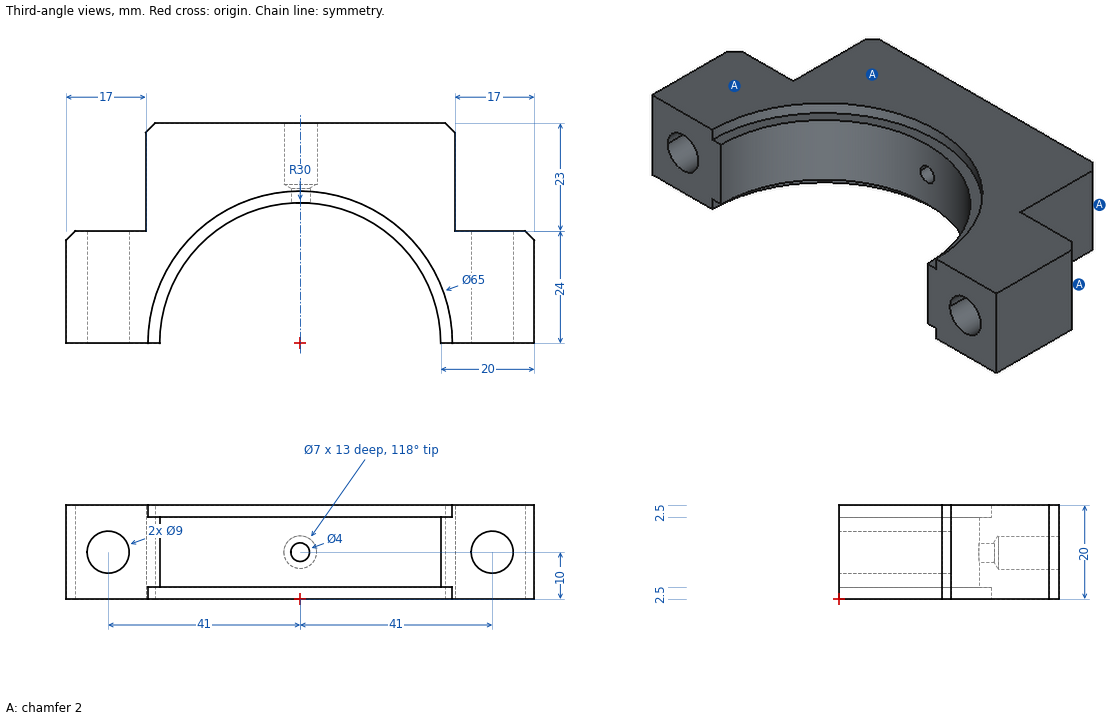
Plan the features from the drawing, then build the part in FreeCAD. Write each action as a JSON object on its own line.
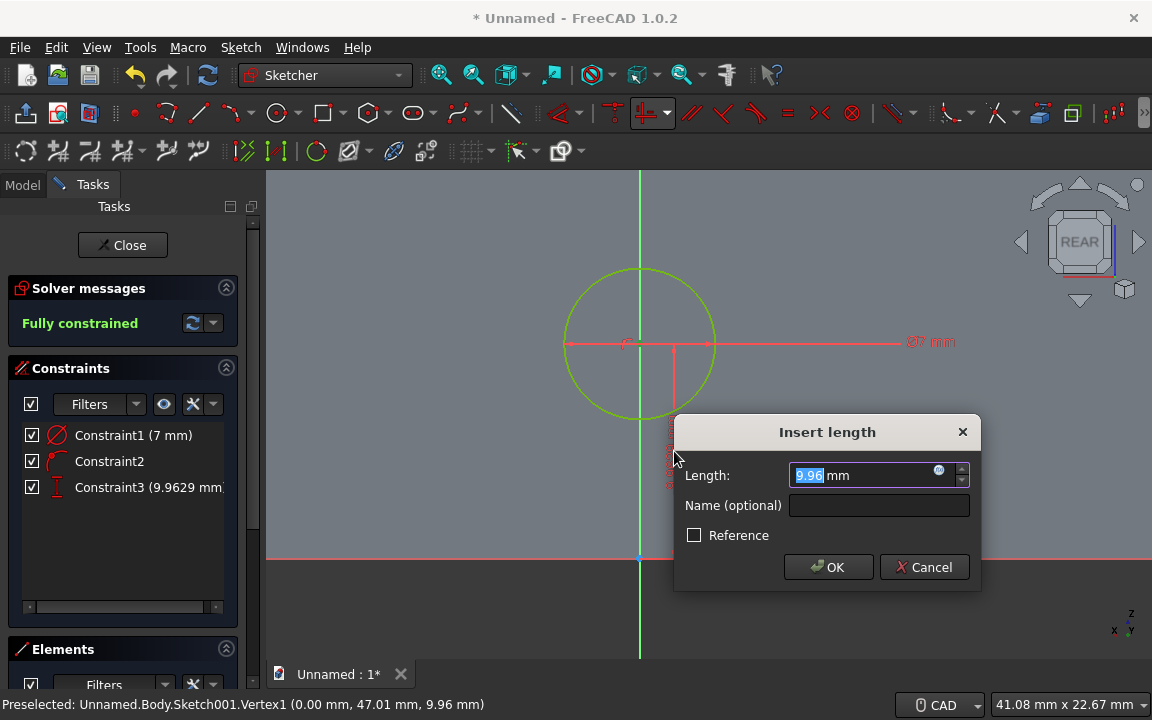
{"action": "type", "text": "10"}
{"action": "key", "text": "Return"}
{"action": "key", "text": "Escape"}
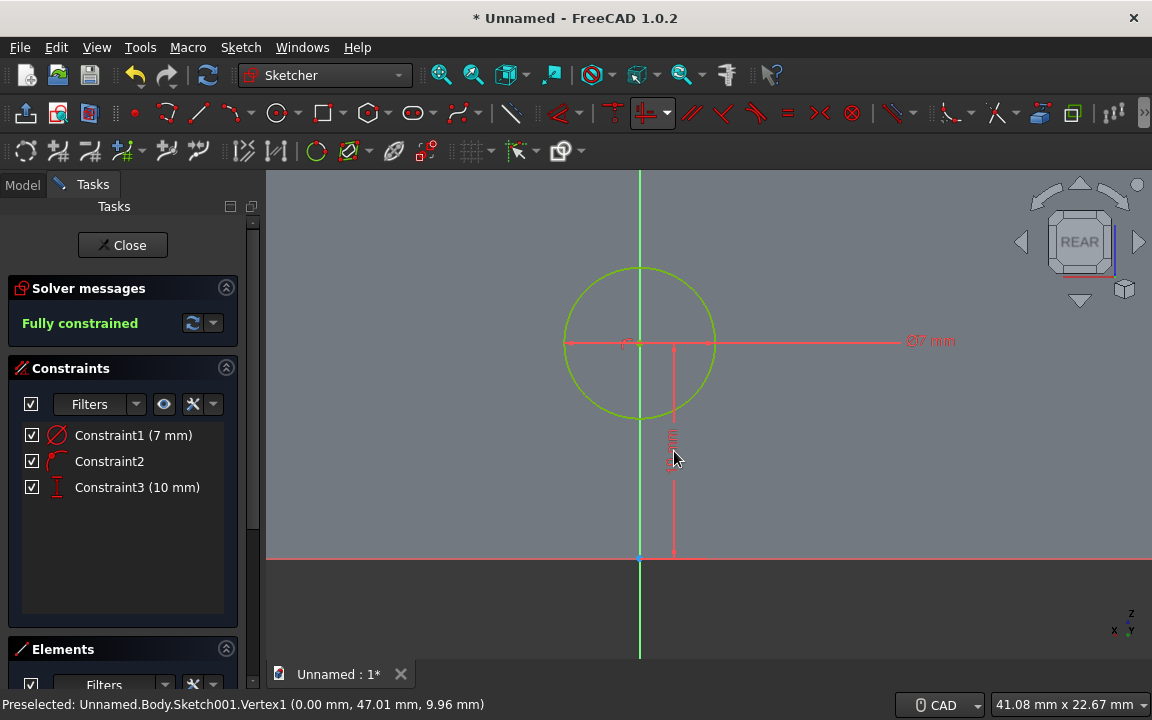
{"action": "left_click", "coordinate": [123, 245]}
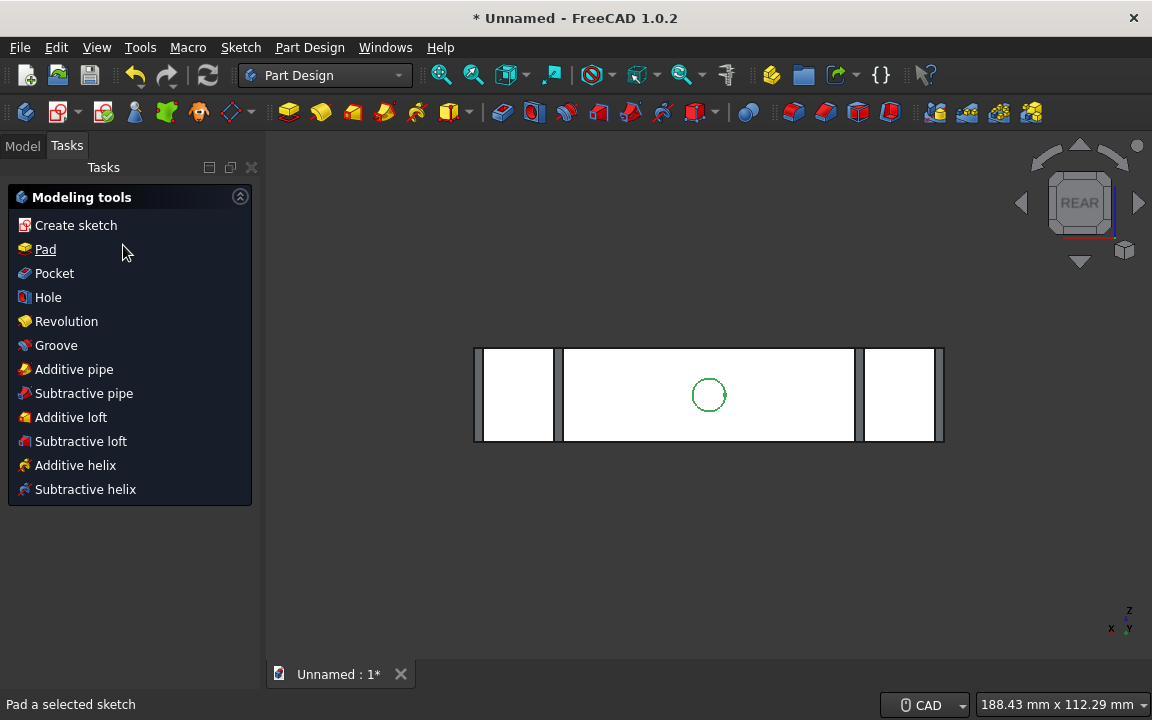
{"action": "left_click", "coordinate": [536, 112]}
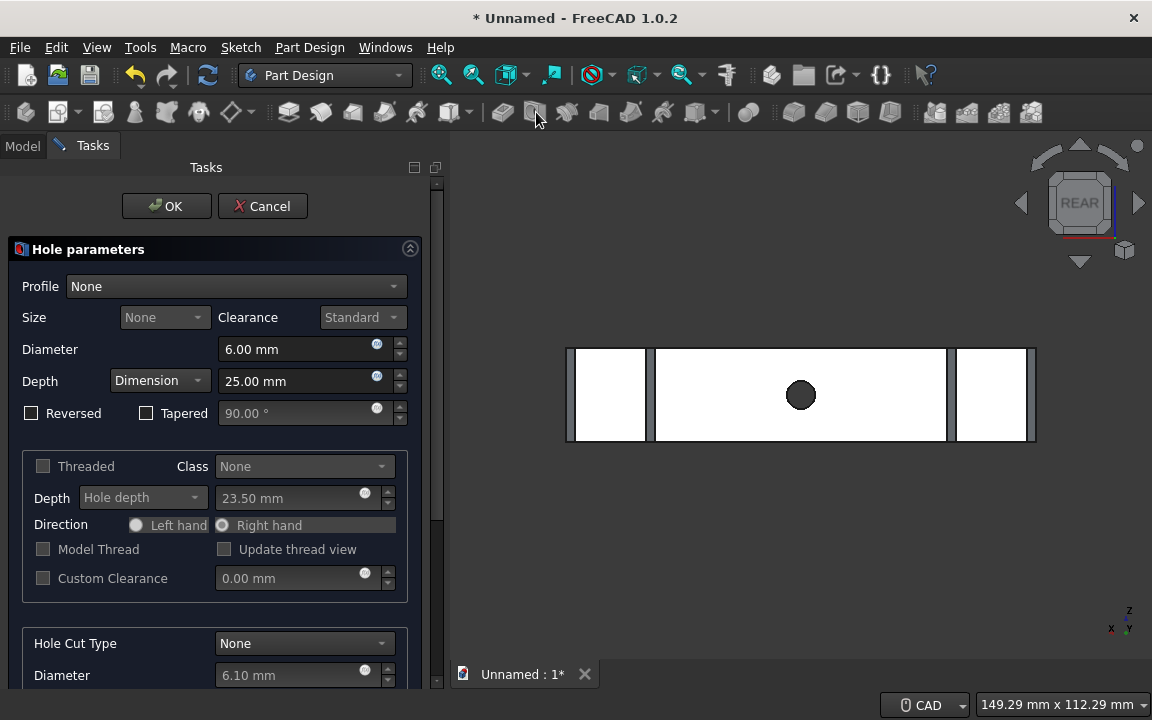
{"action": "triple_click", "coordinate": [305, 349]}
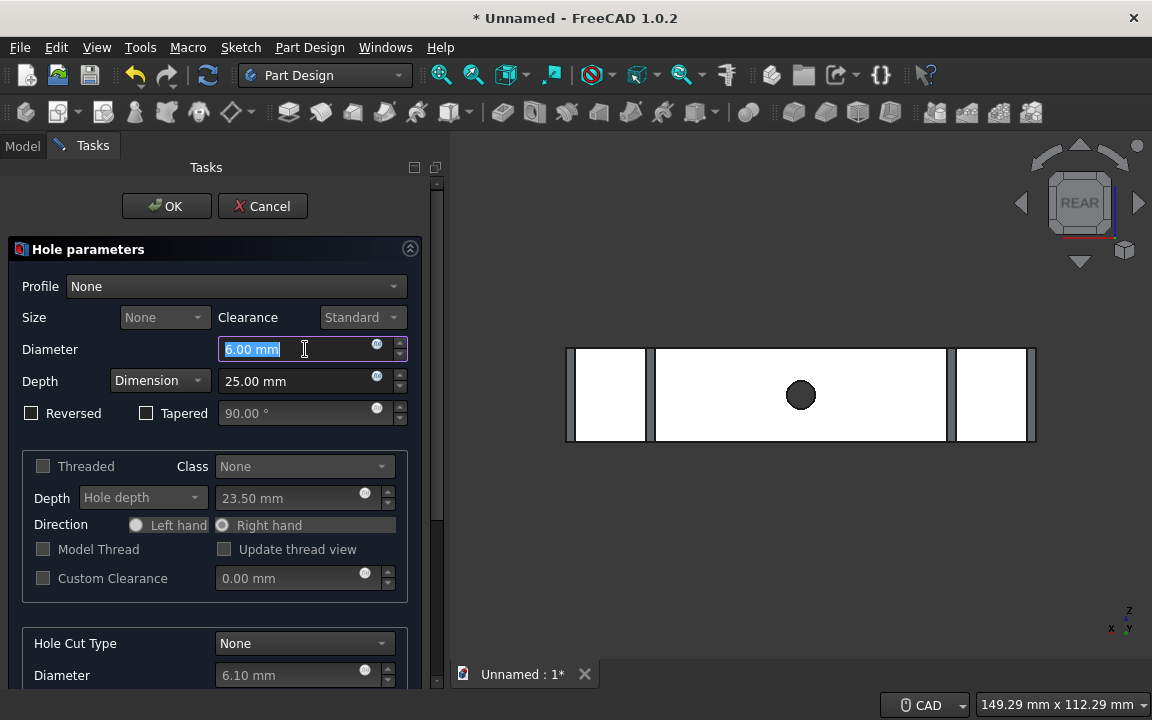
{"action": "type", "text": "7"}
{"action": "key", "text": "Tab"}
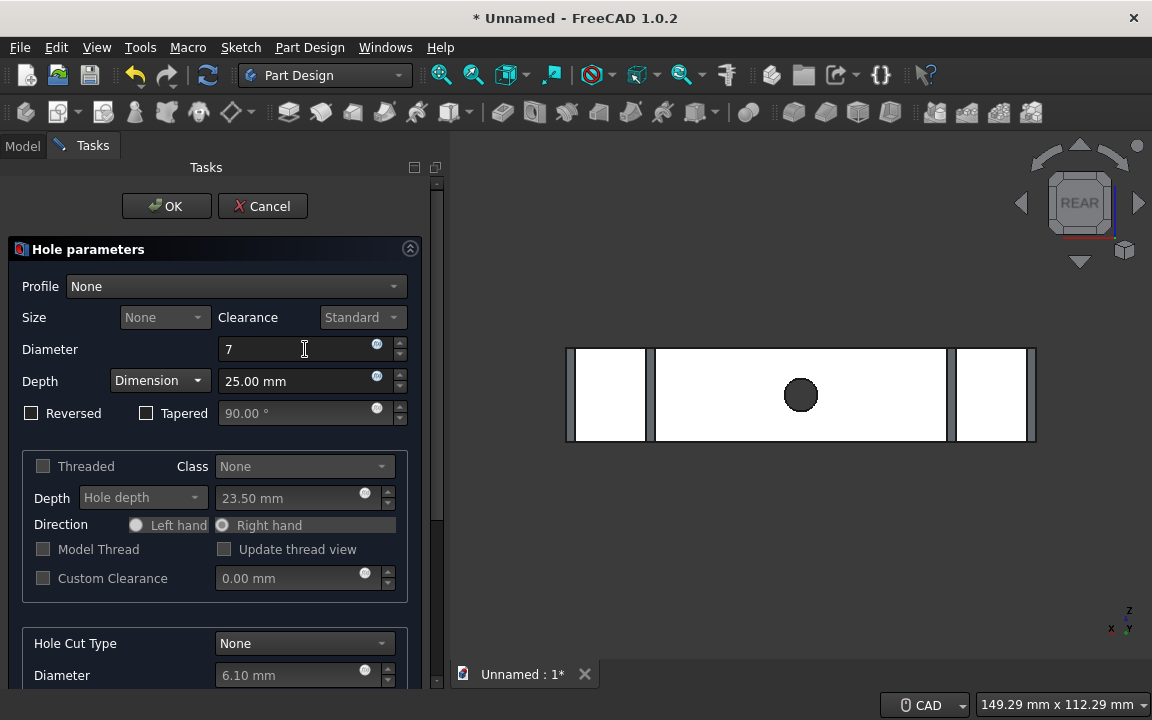
{"action": "triple_click", "coordinate": [305, 381]}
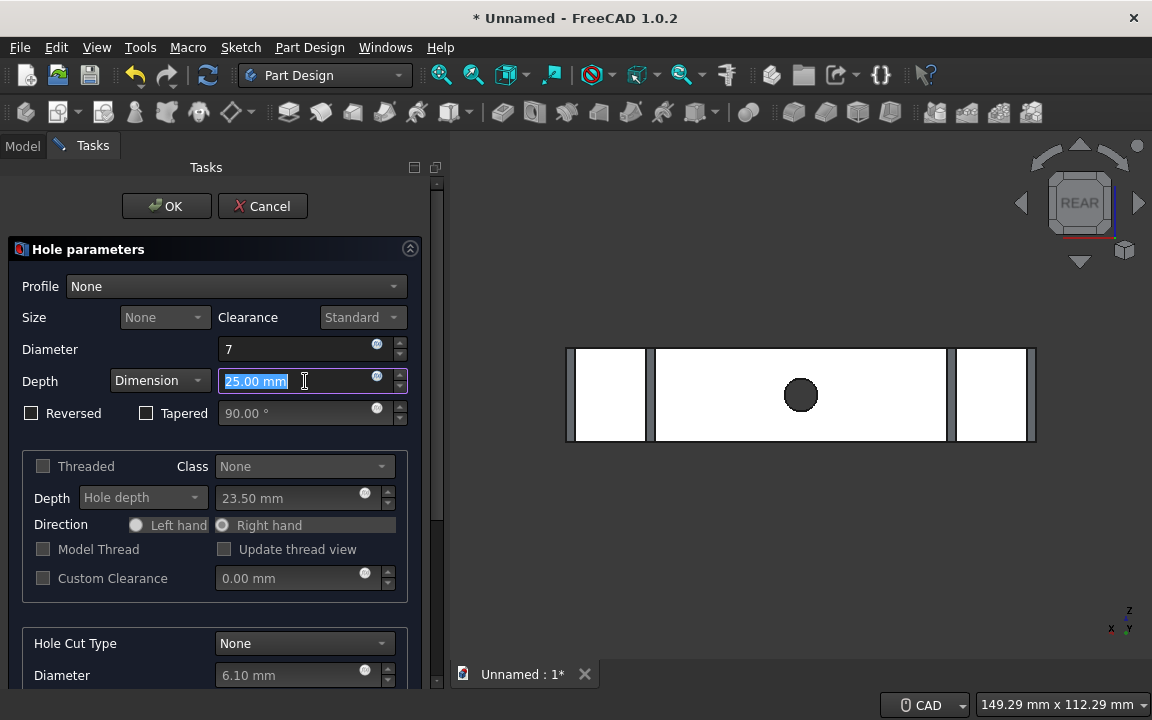
{"action": "type", "text": "13"}
{"action": "key", "text": "Tab"}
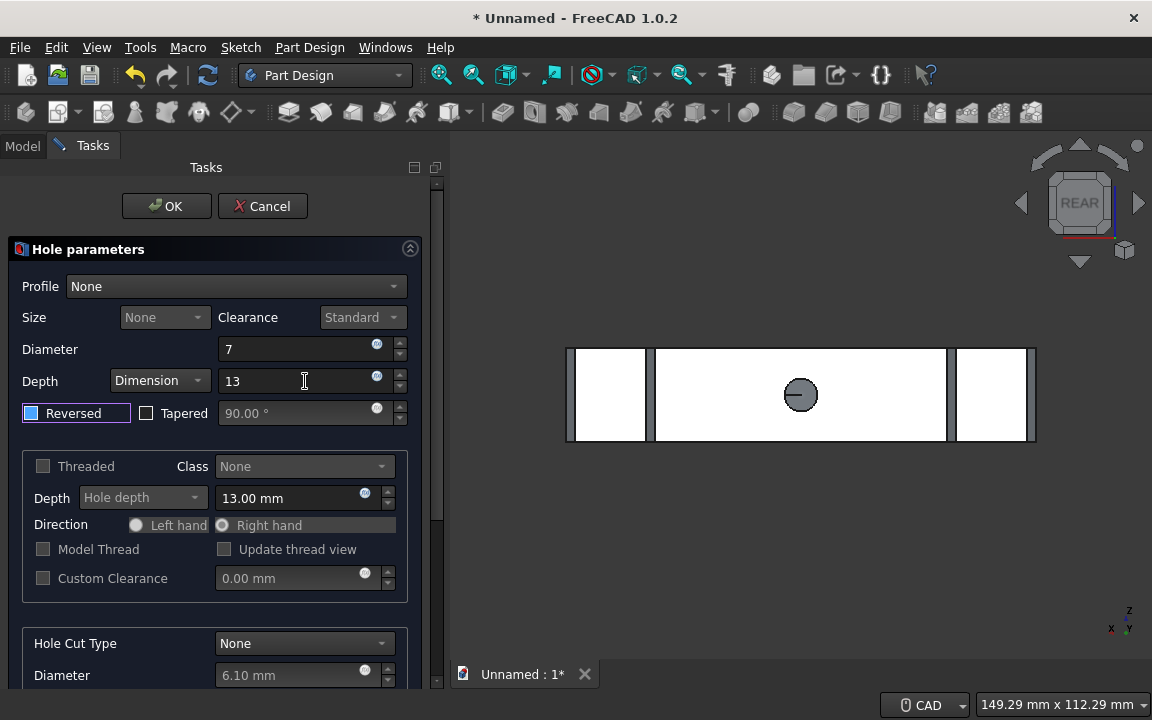
{"action": "left_click", "coordinate": [167, 206]}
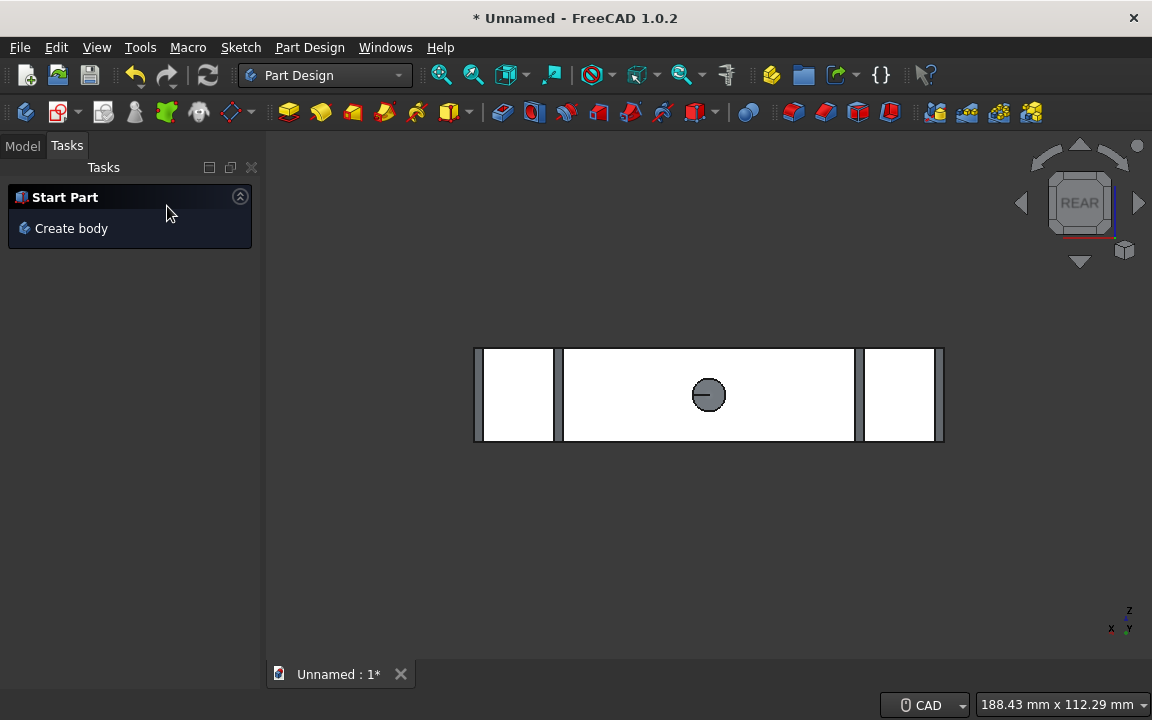
{"action": "left_click", "coordinate": [519, 394]}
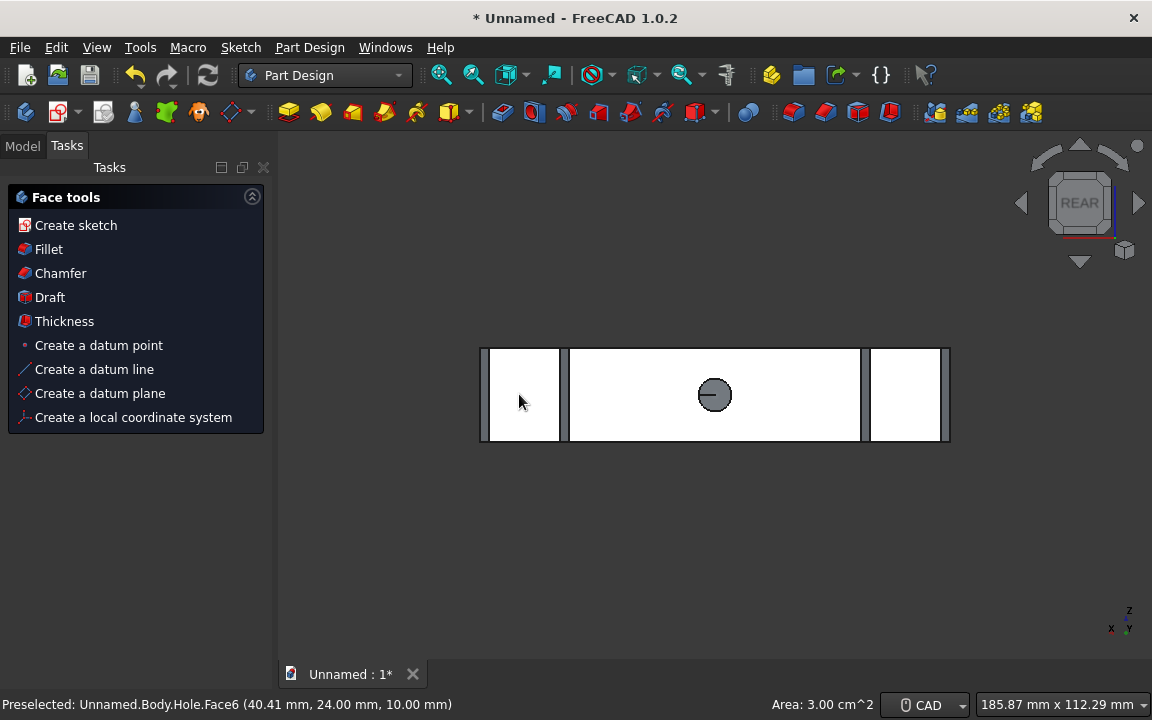
{"action": "left_click", "coordinate": [58, 112]}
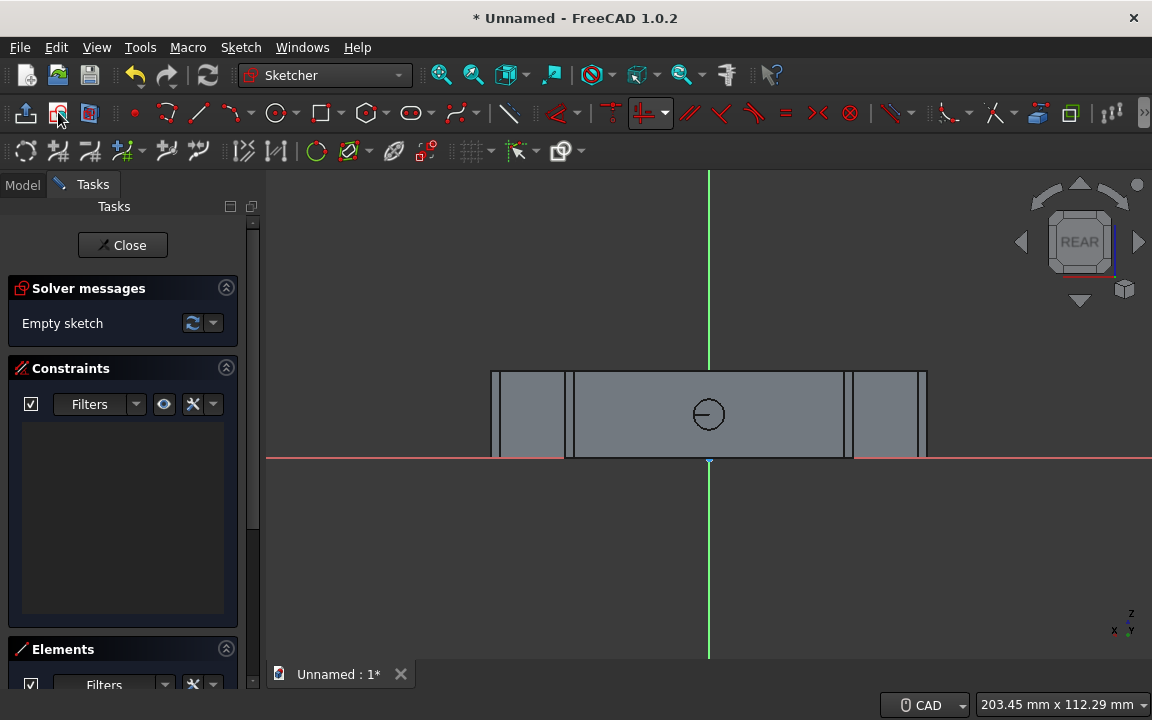
{"action": "left_click", "coordinate": [276, 114]}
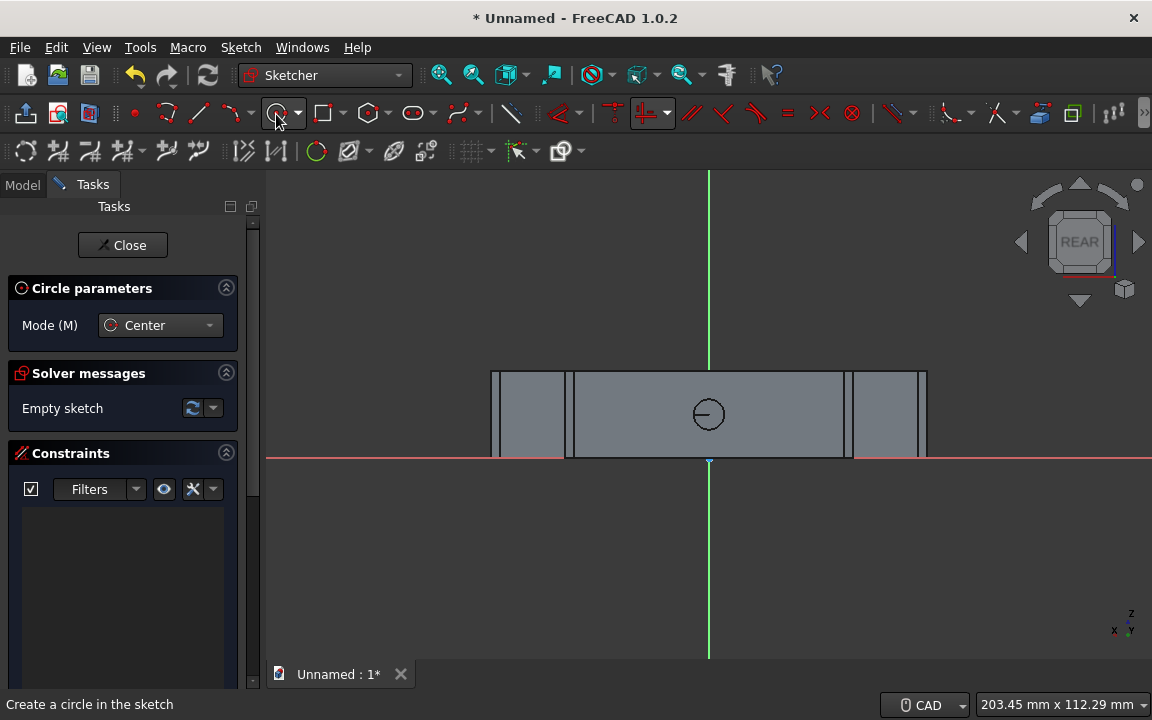
{"action": "left_click", "coordinate": [888, 415]}
{"action": "mouse_move", "coordinate": [901, 401]}